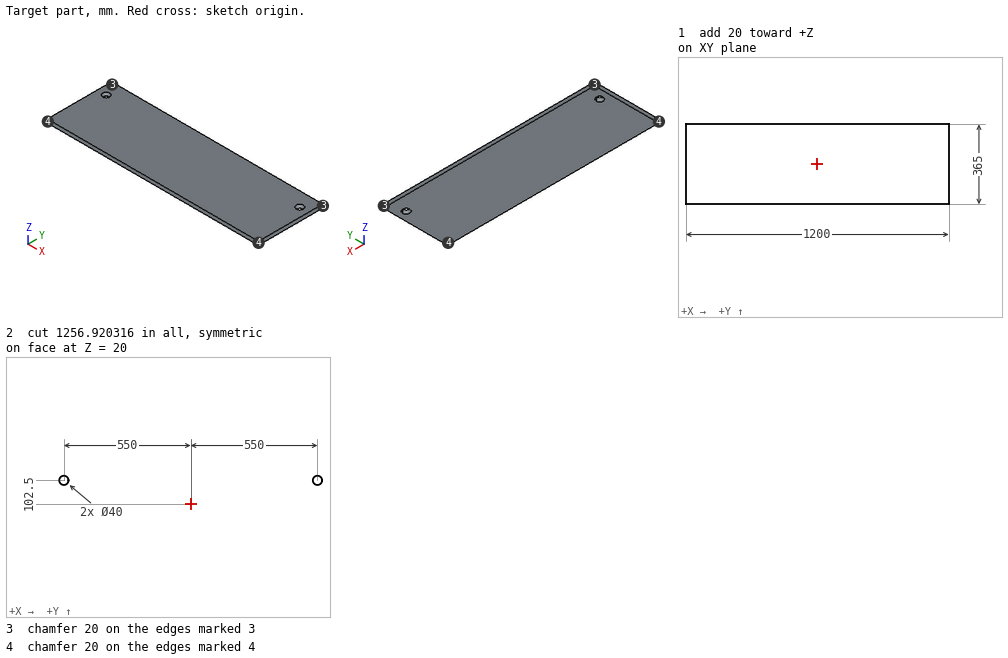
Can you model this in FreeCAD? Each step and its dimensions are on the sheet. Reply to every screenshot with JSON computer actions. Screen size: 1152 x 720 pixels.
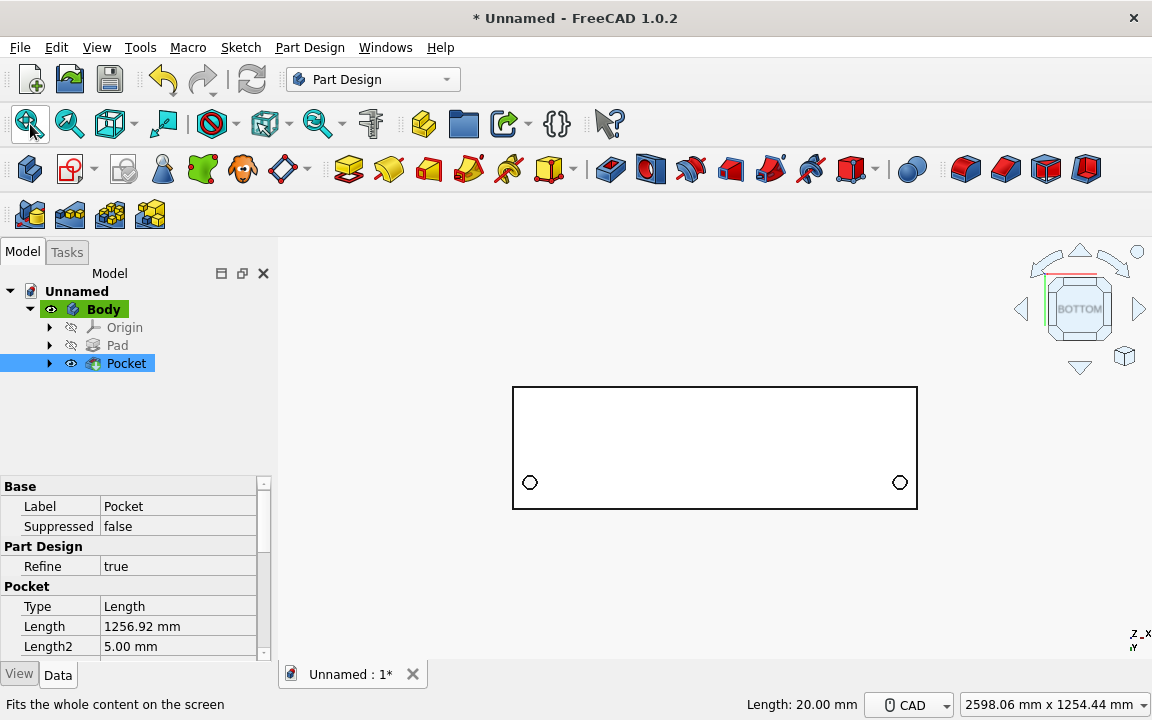
{"action": "key", "text": "4"}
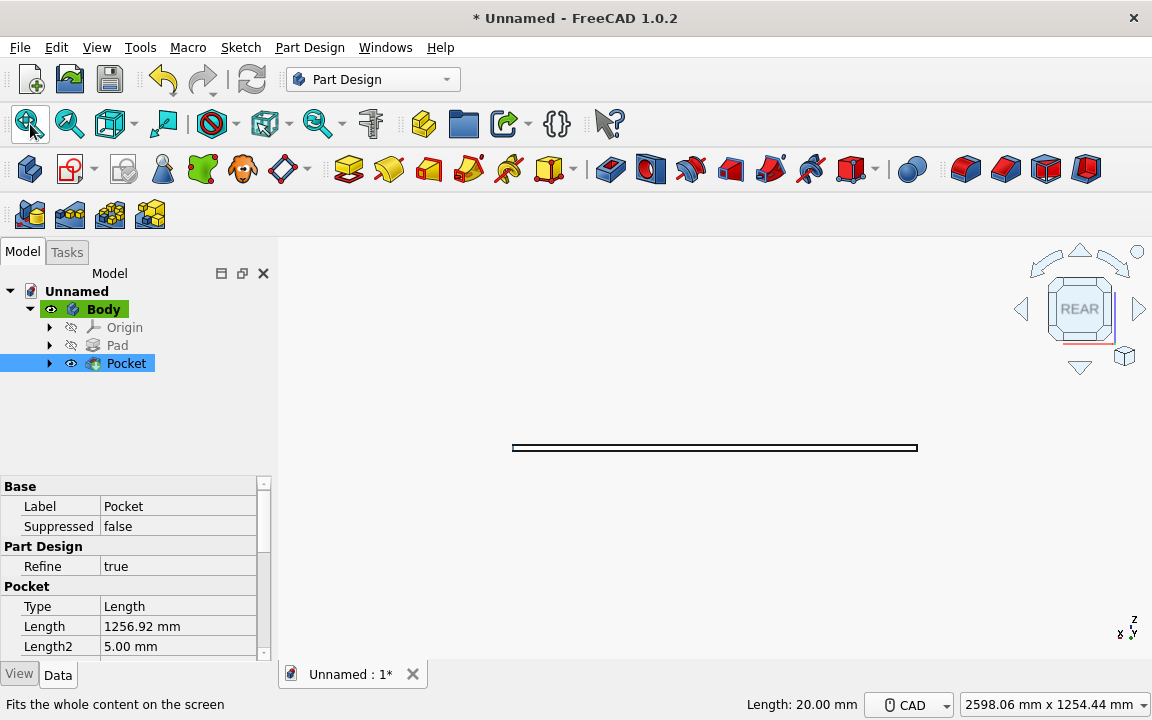
{"action": "scroll", "coordinate": [917, 447], "scroll_direction": "up", "scroll_amount": 9}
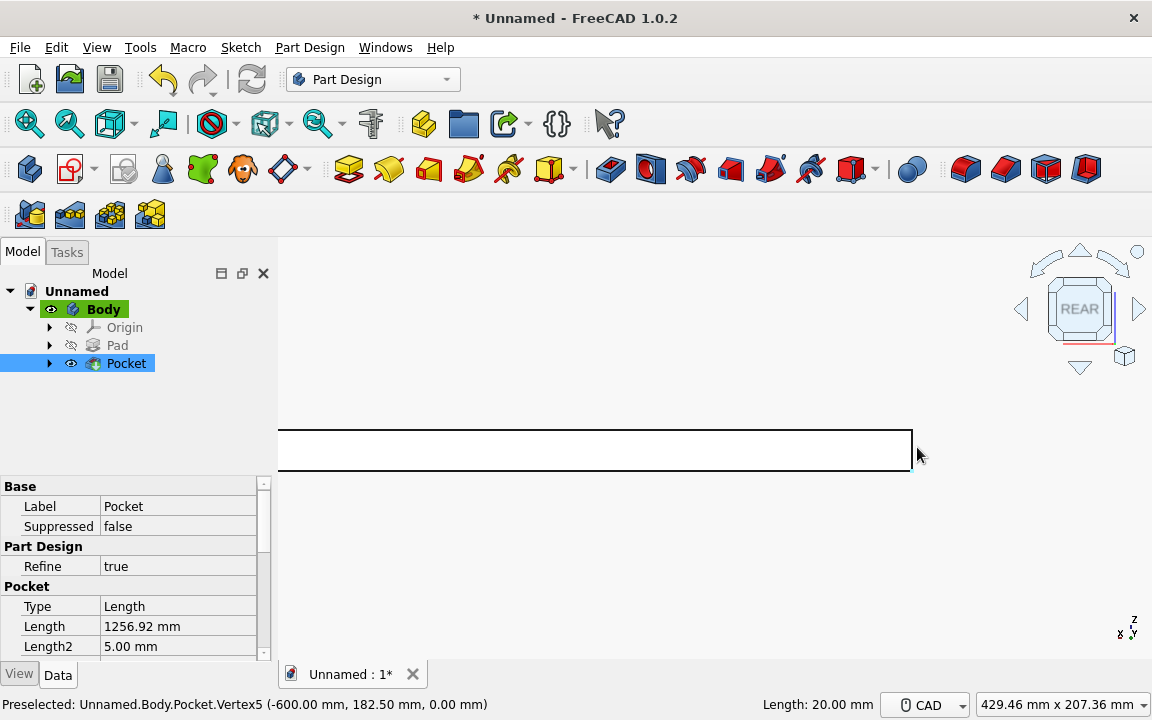
{"action": "left_click", "coordinate": [912, 450], "text": "ctrl"}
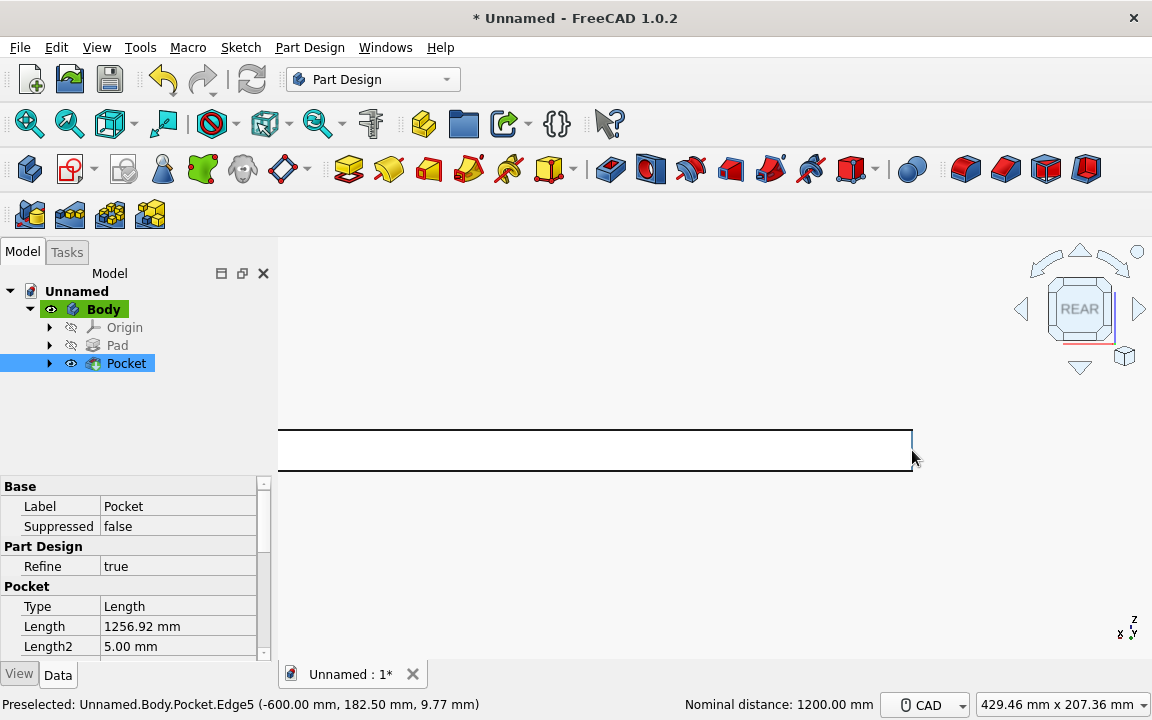
{"action": "left_click", "coordinate": [1006, 170]}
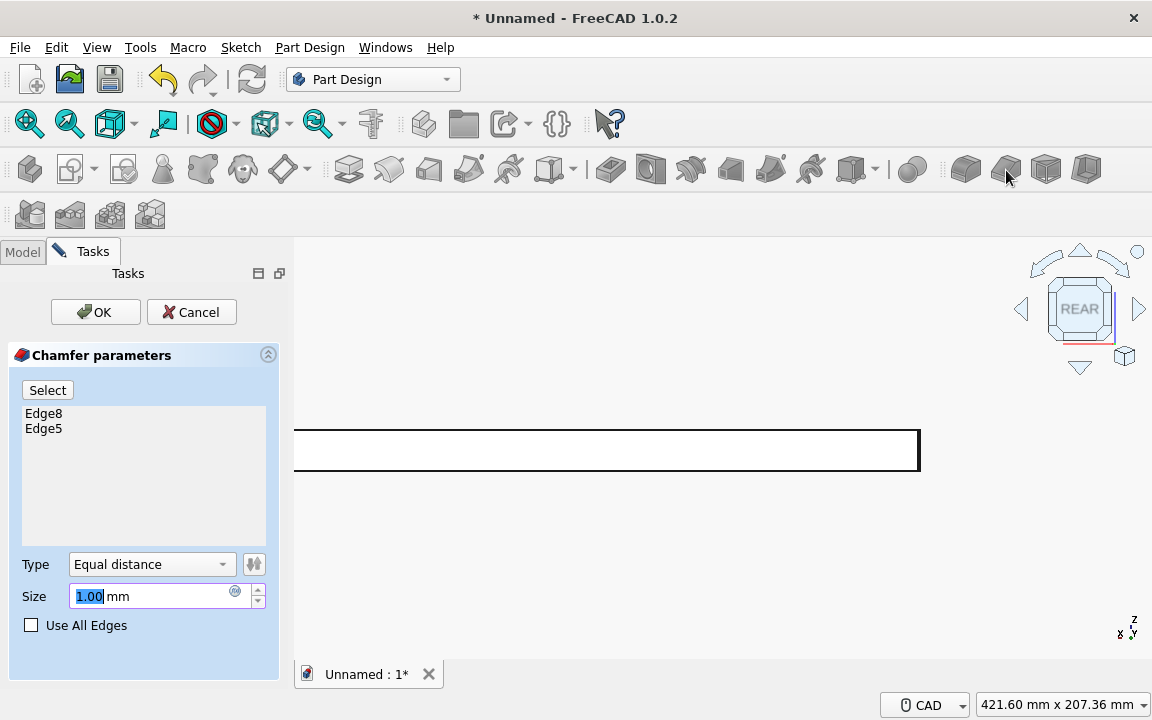
{"action": "type", "text": "20"}
{"action": "key", "text": "Tab"}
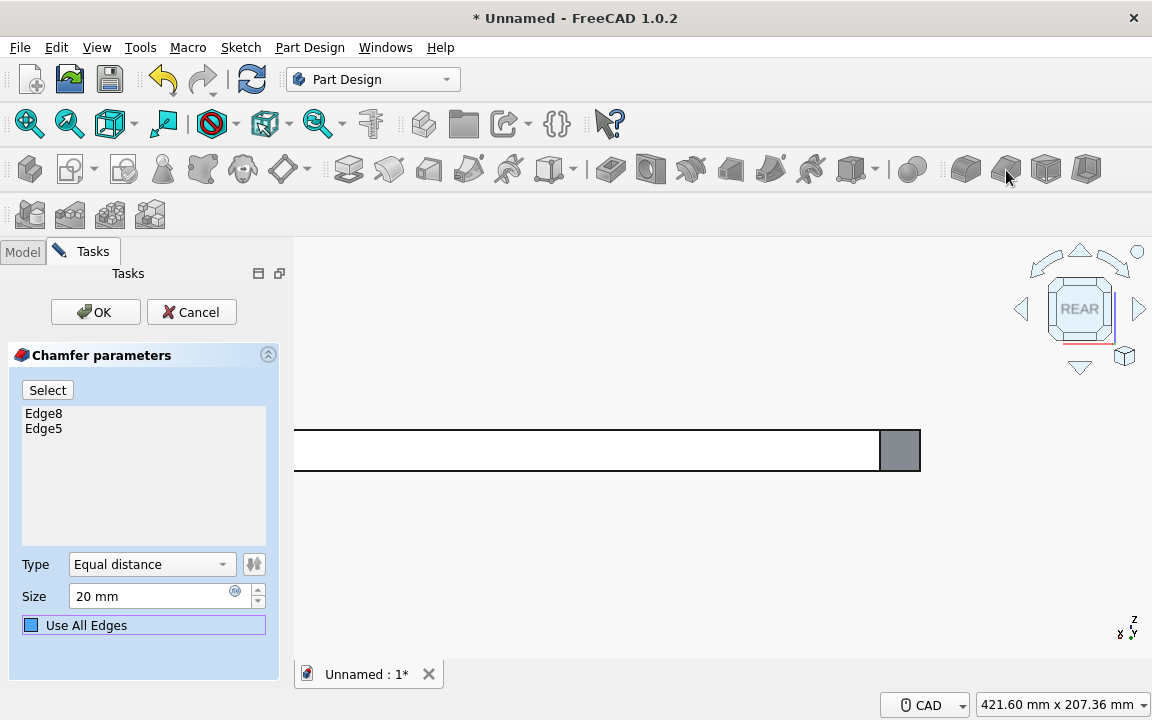
{"action": "left_click", "coordinate": [96, 312]}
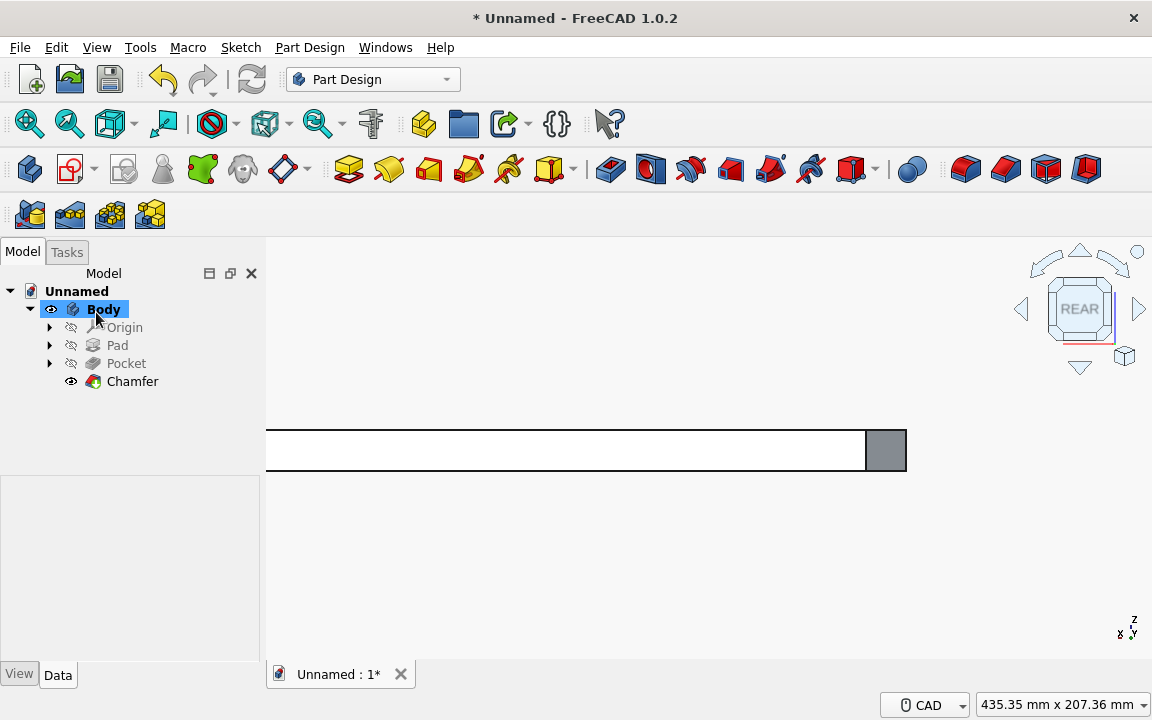
{"action": "left_click", "coordinate": [30, 124]}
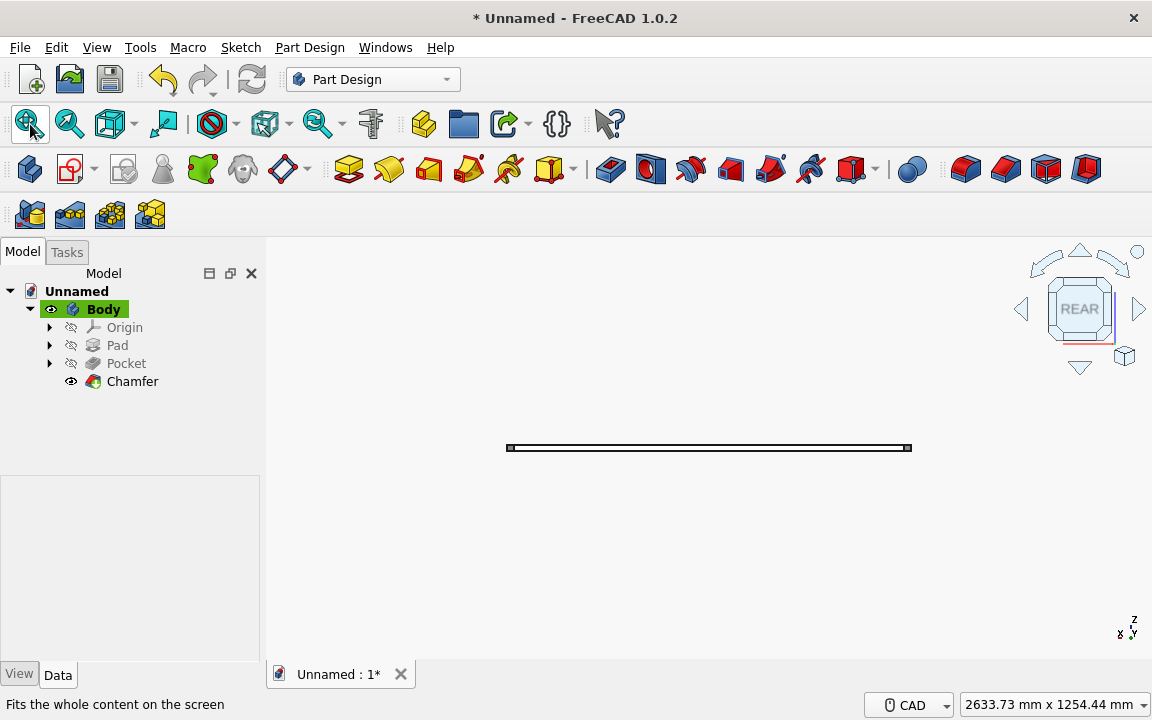
{"action": "scroll", "coordinate": [507, 447], "scroll_direction": "up", "scroll_amount": 9}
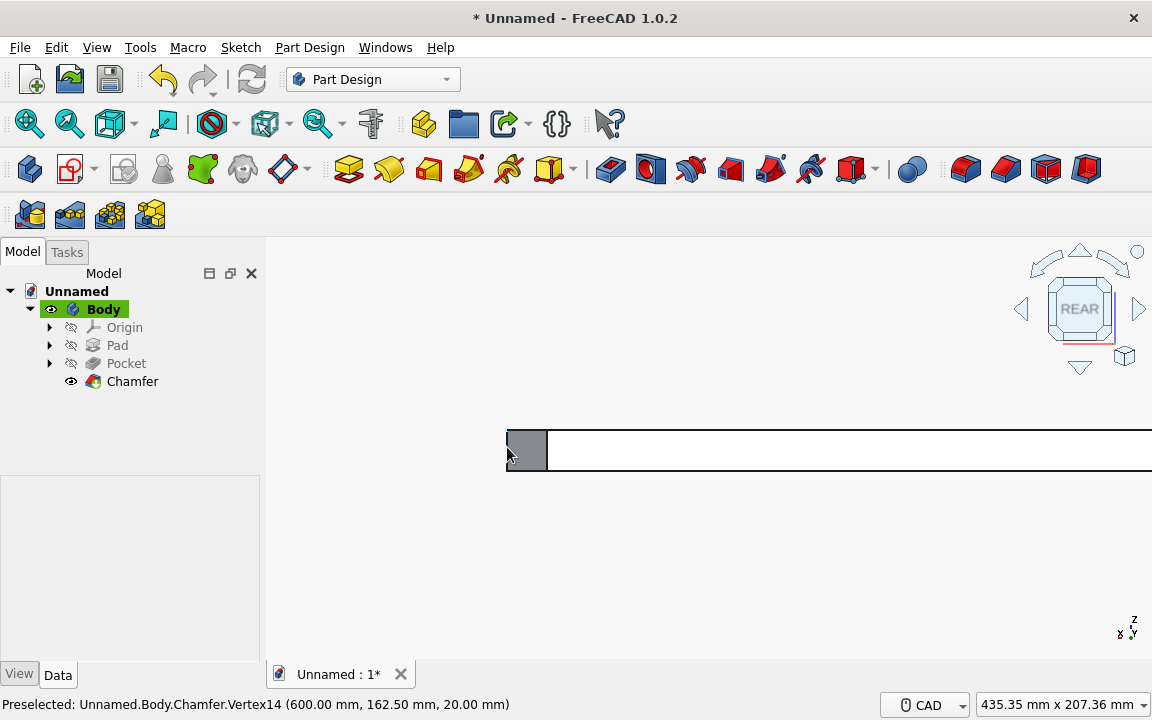
{"action": "key", "text": "v f"}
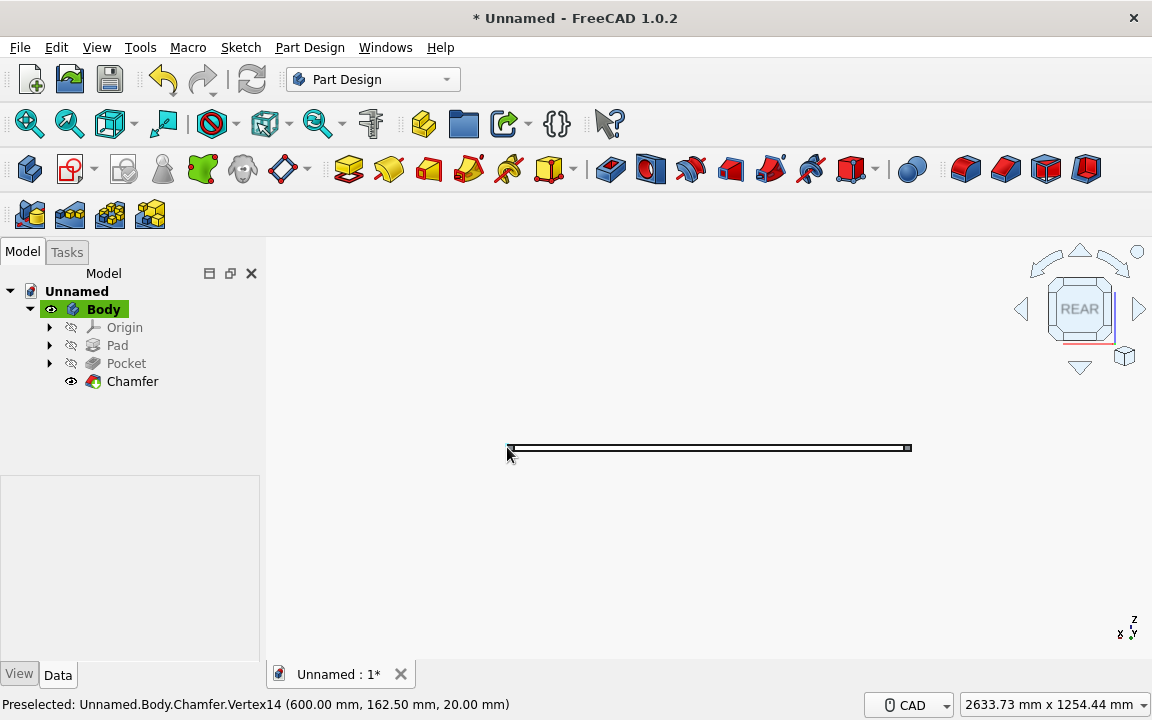
{"action": "key", "text": "0"}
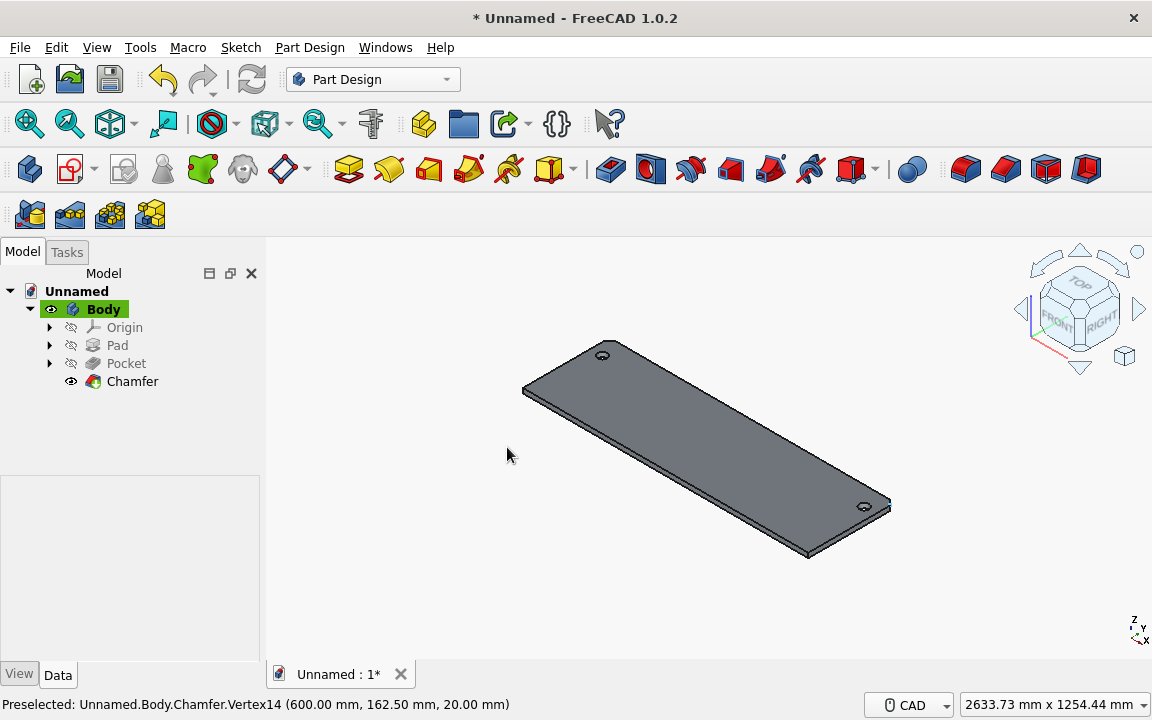
{"action": "scroll", "coordinate": [808, 554], "scroll_direction": "up", "scroll_amount": 9}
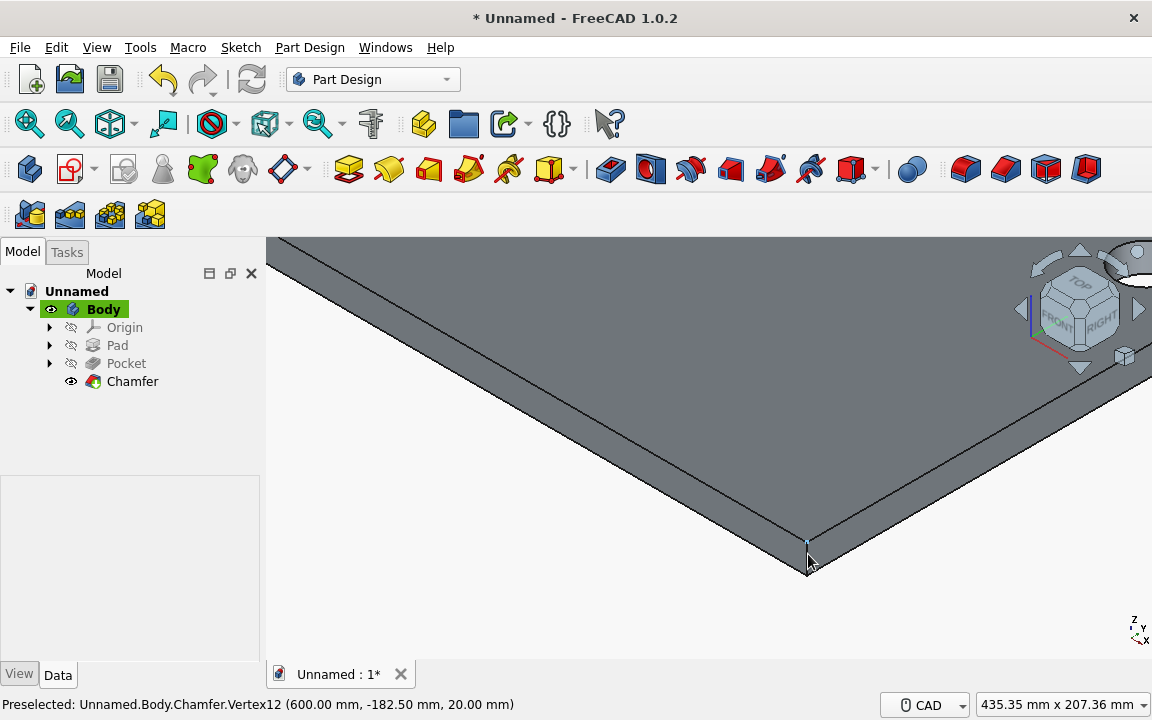
{"action": "left_click", "coordinate": [807, 558]}